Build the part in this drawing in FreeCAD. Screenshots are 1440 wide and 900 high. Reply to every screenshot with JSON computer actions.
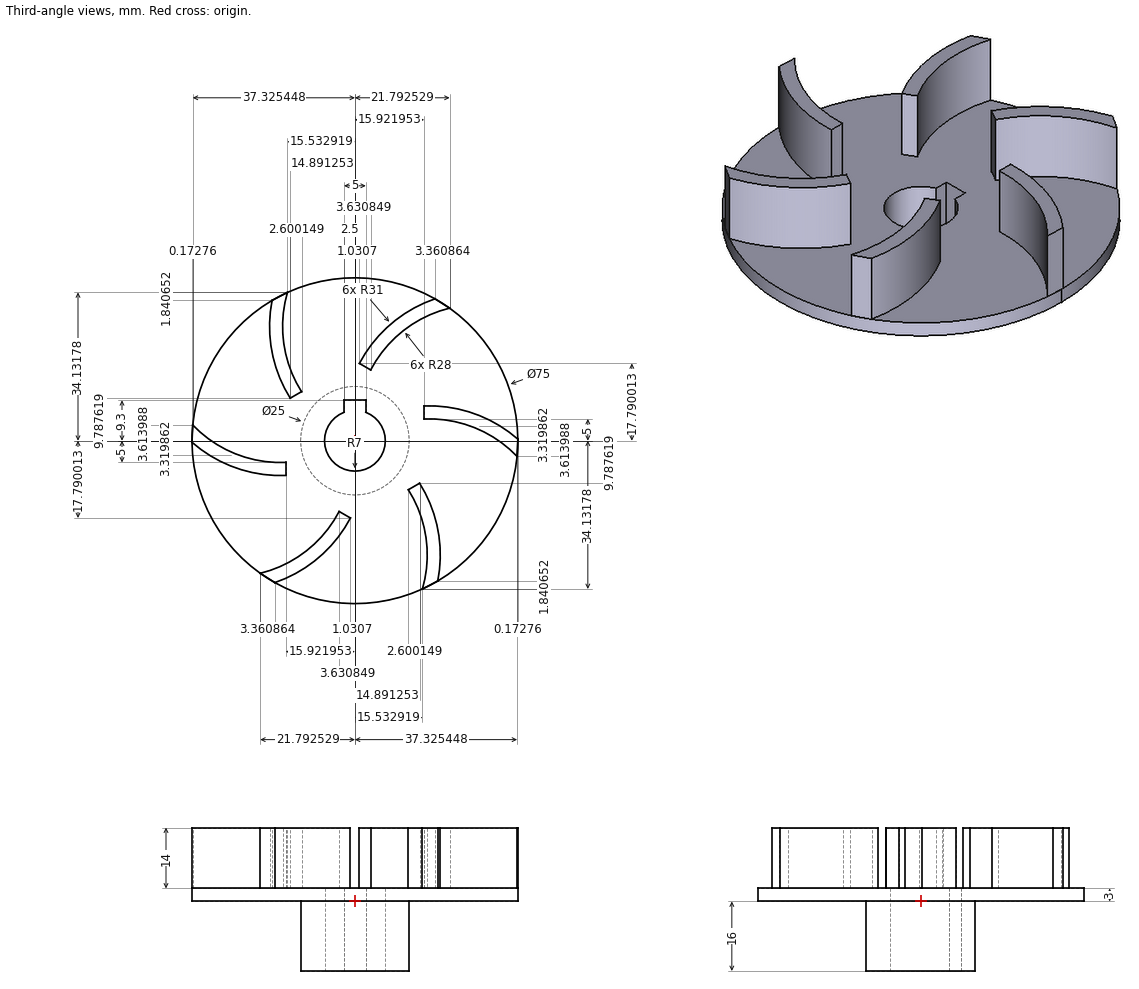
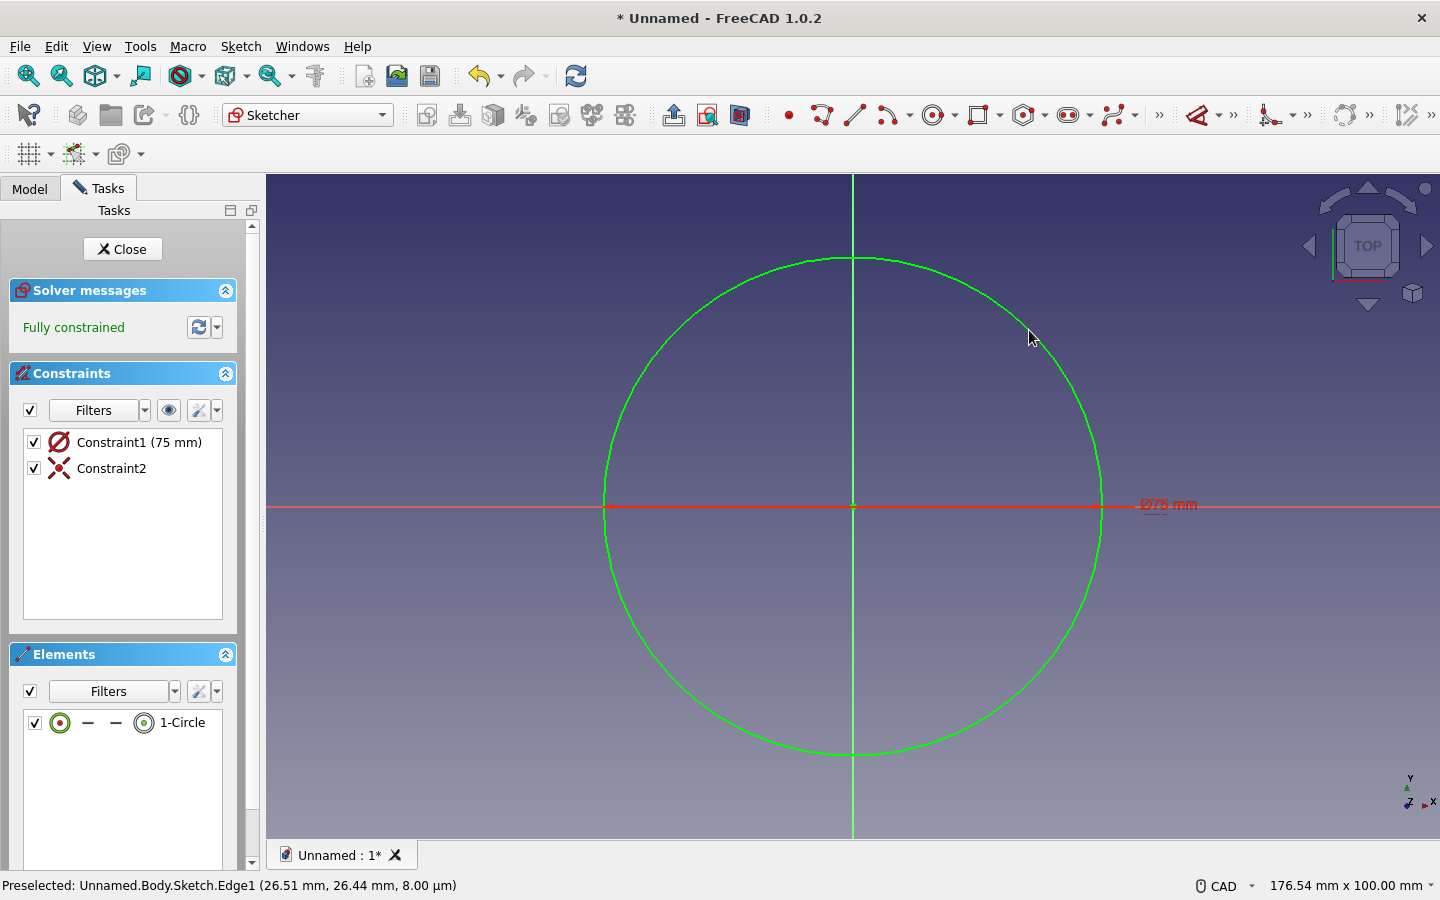
{"action": "left_click", "coordinate": [123, 249]}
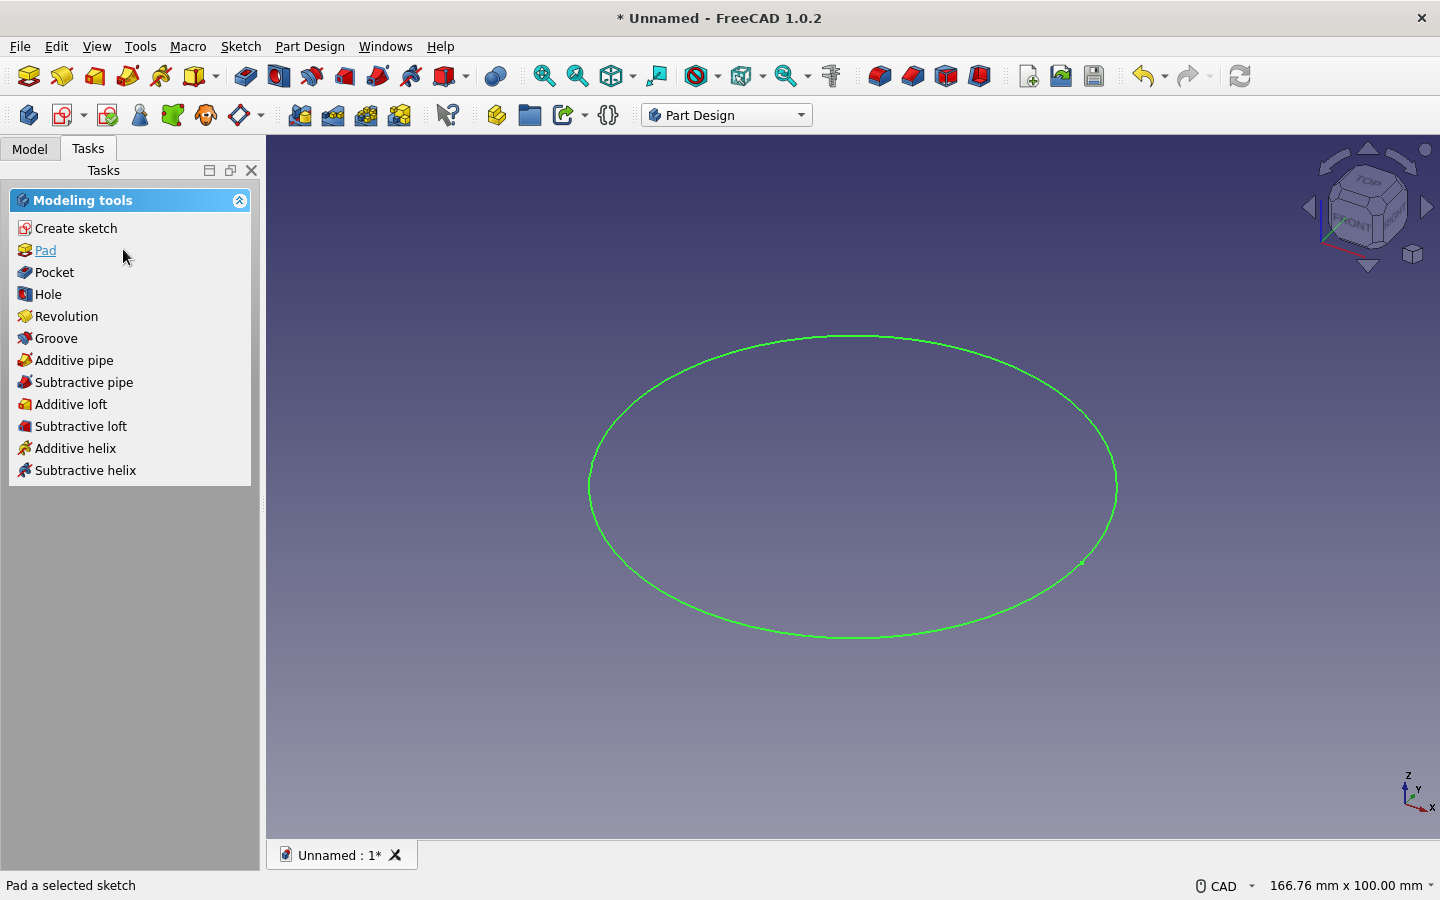
{"action": "left_click", "coordinate": [29, 76]}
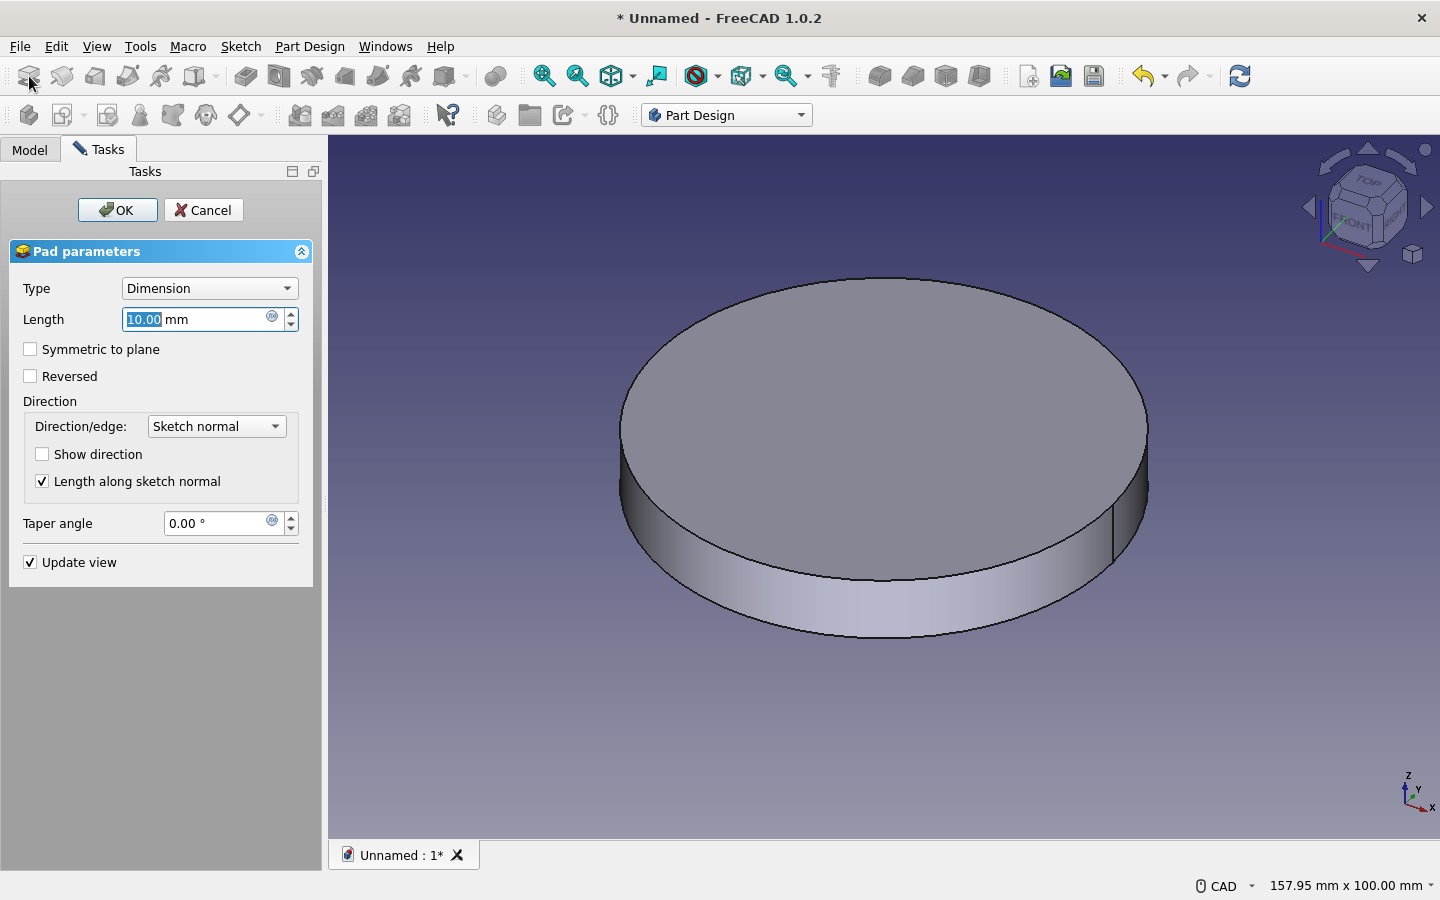
{"action": "type", "text": "3"}
{"action": "key", "text": "Tab"}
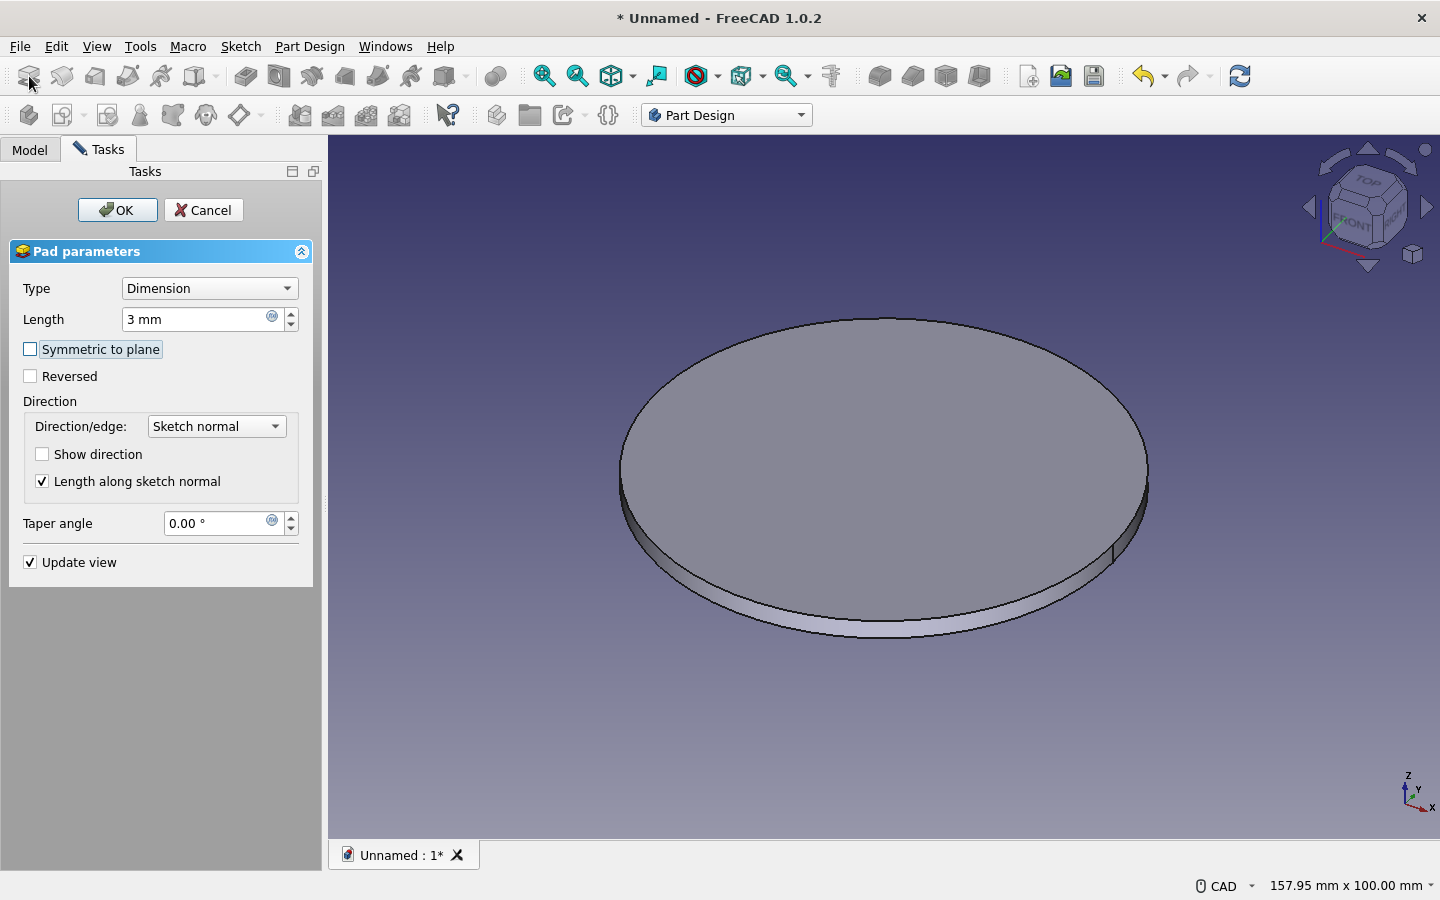
{"action": "left_click", "coordinate": [118, 210]}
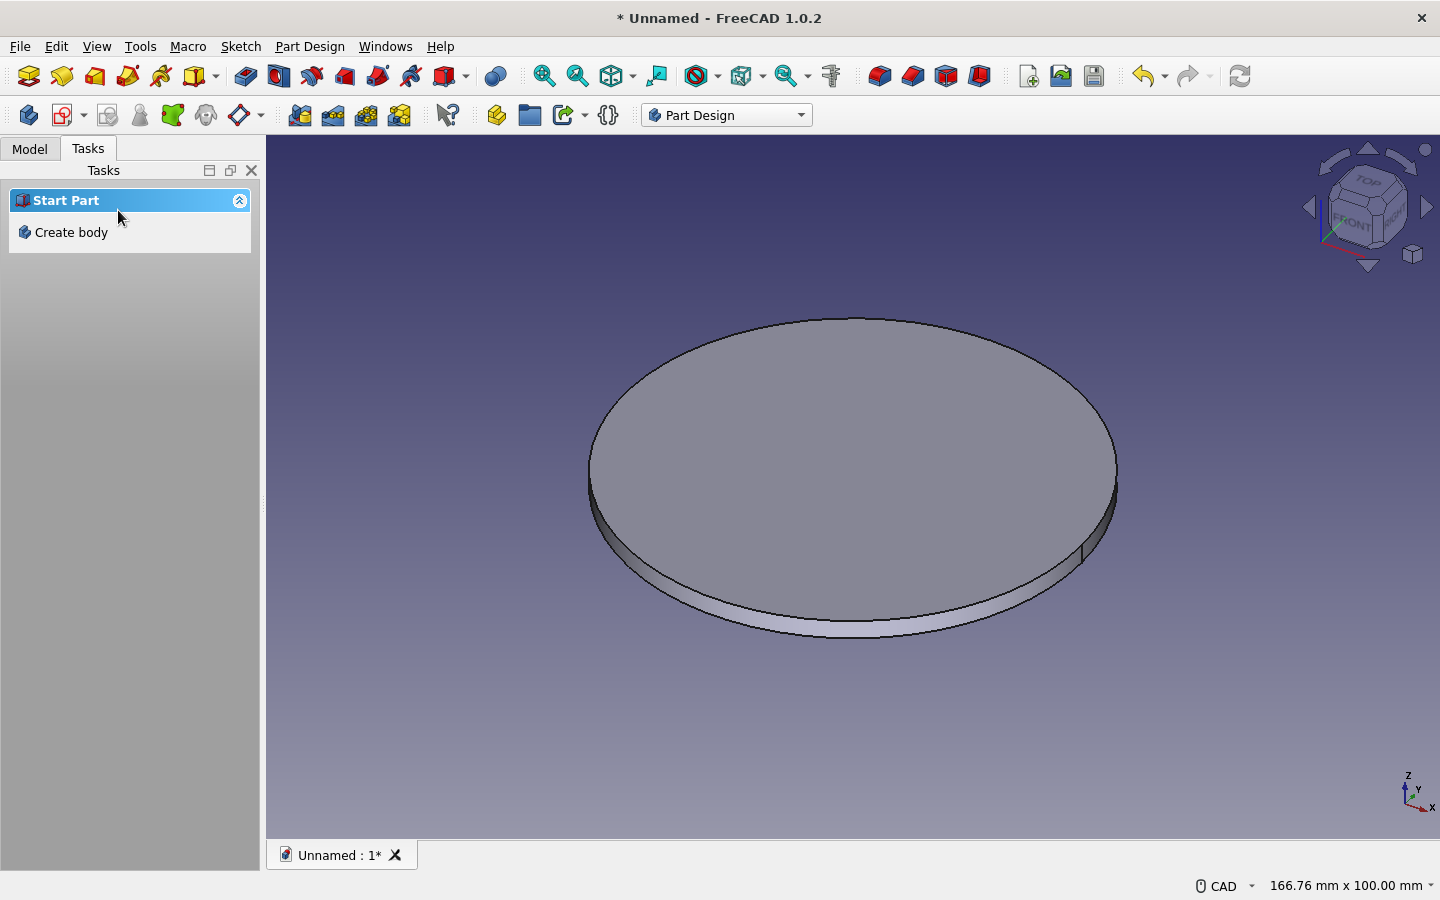
{"action": "left_click", "coordinate": [853, 469]}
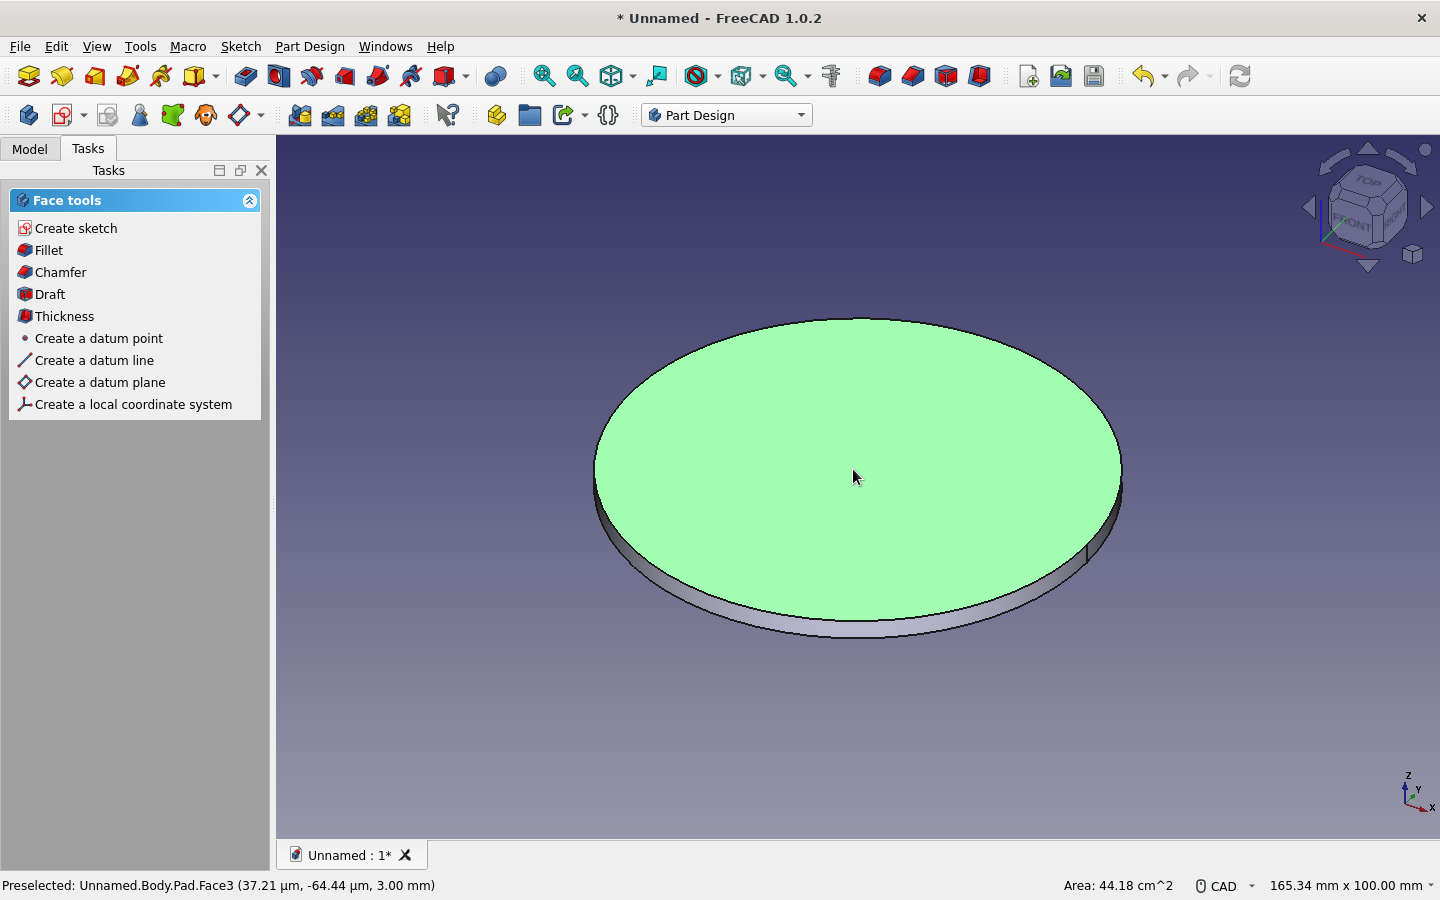
{"action": "left_click", "coordinate": [62, 116]}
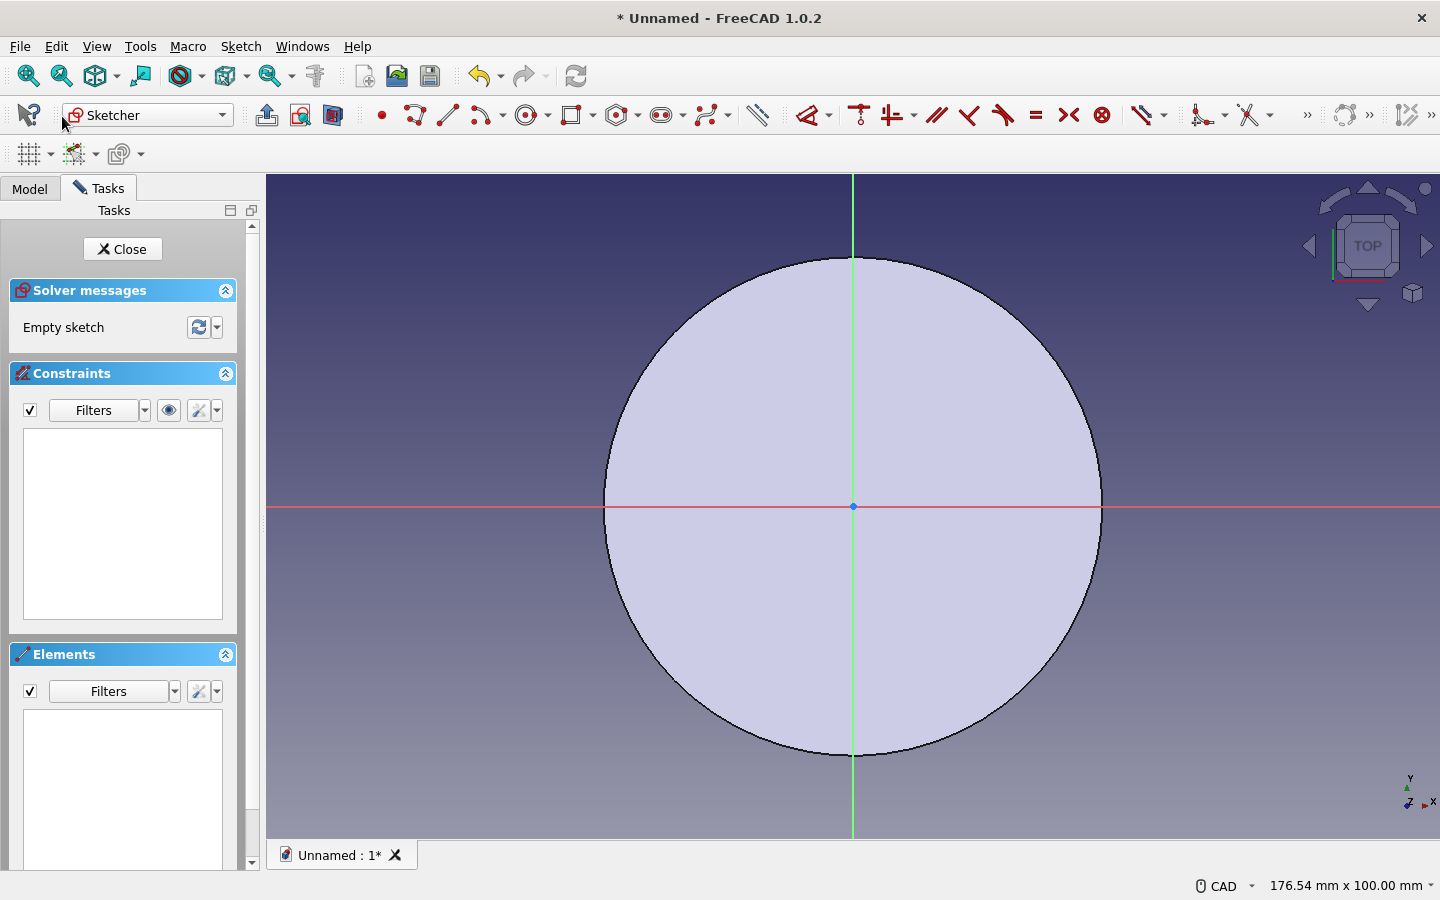
{"action": "key", "text": "g l"}